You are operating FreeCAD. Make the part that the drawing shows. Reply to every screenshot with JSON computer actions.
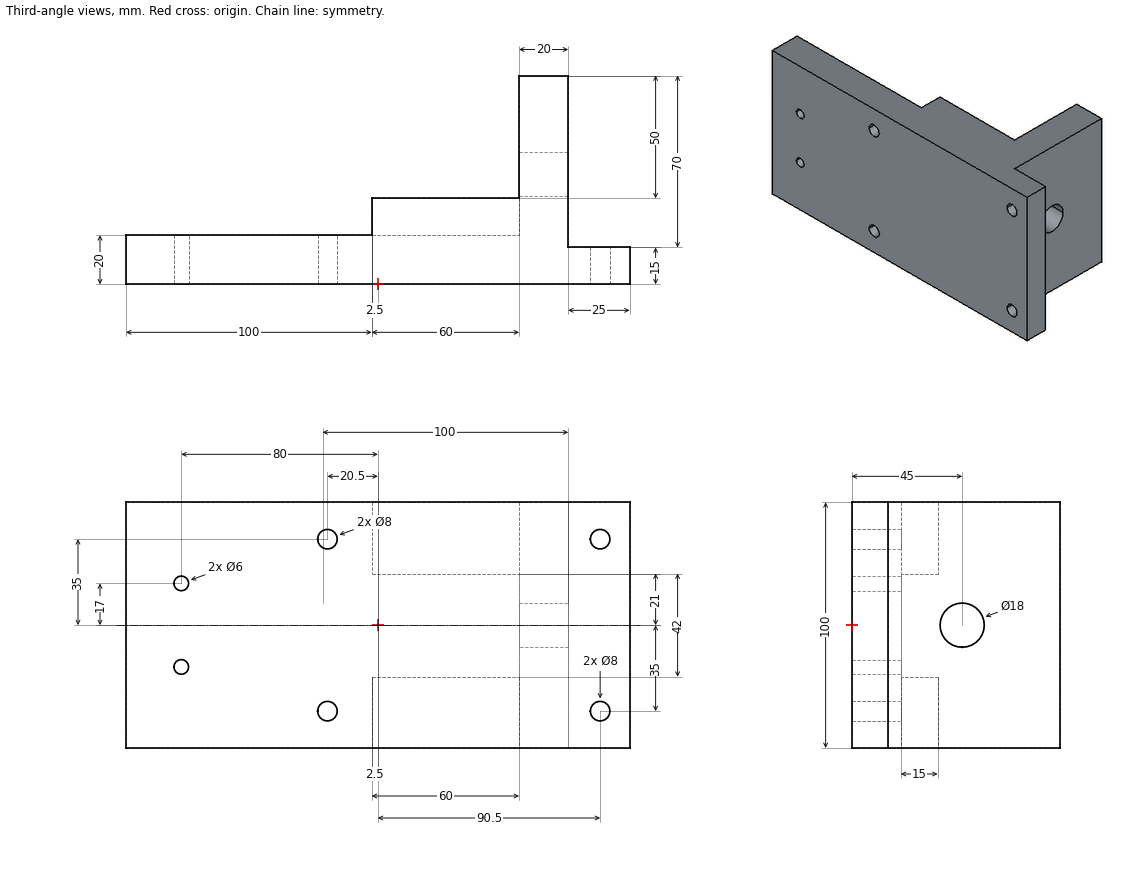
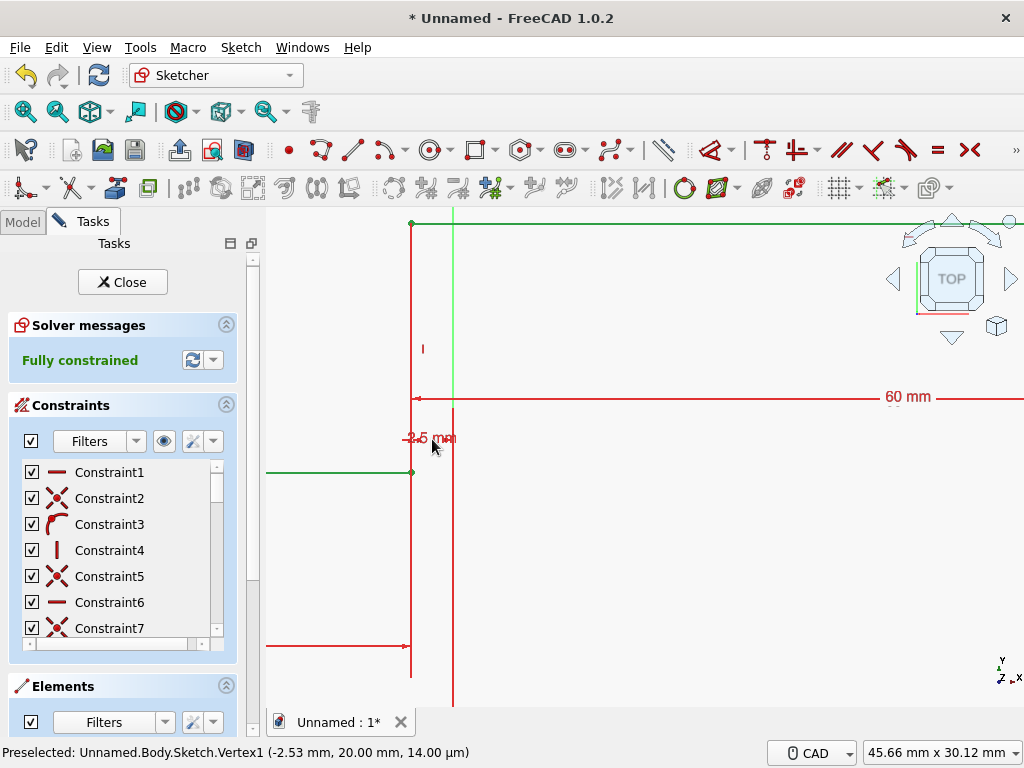
{"action": "left_click", "coordinate": [123, 282]}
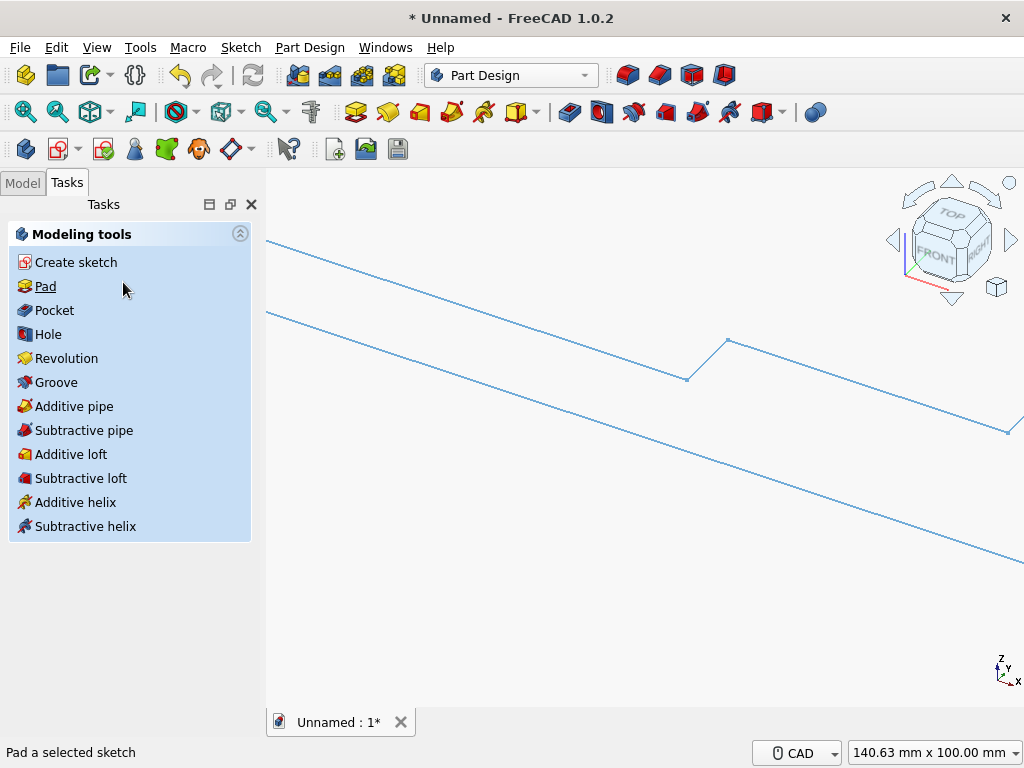
{"action": "left_click", "coordinate": [356, 112]}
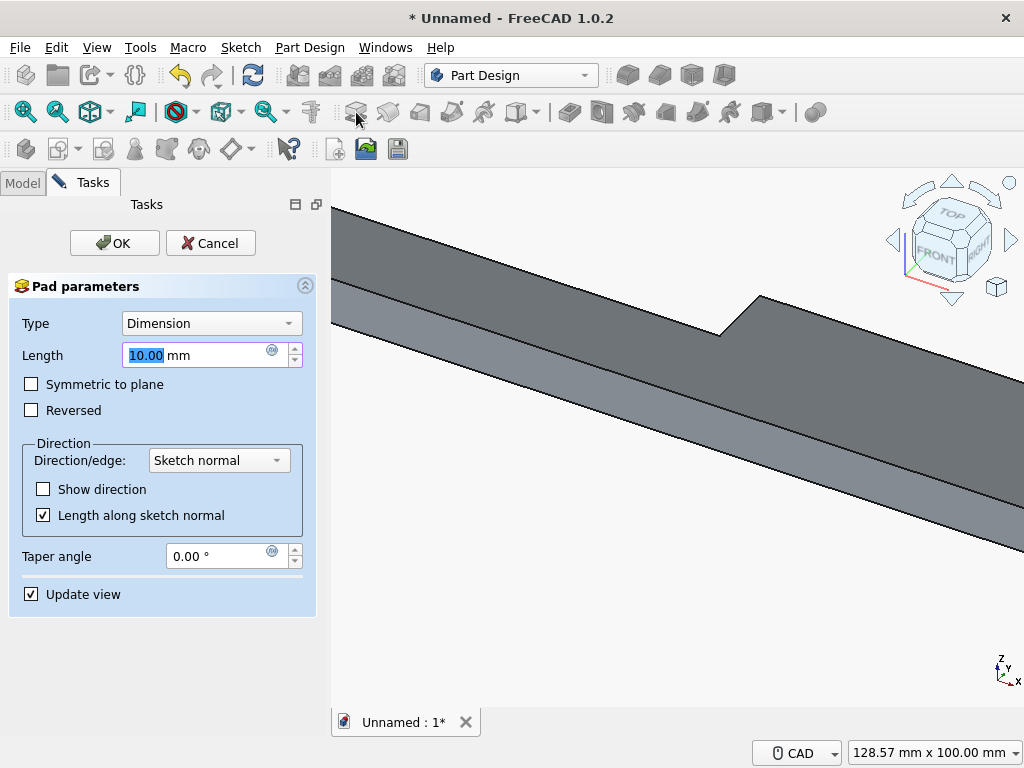
{"action": "type", "text": "100"}
{"action": "key", "text": "Tab"}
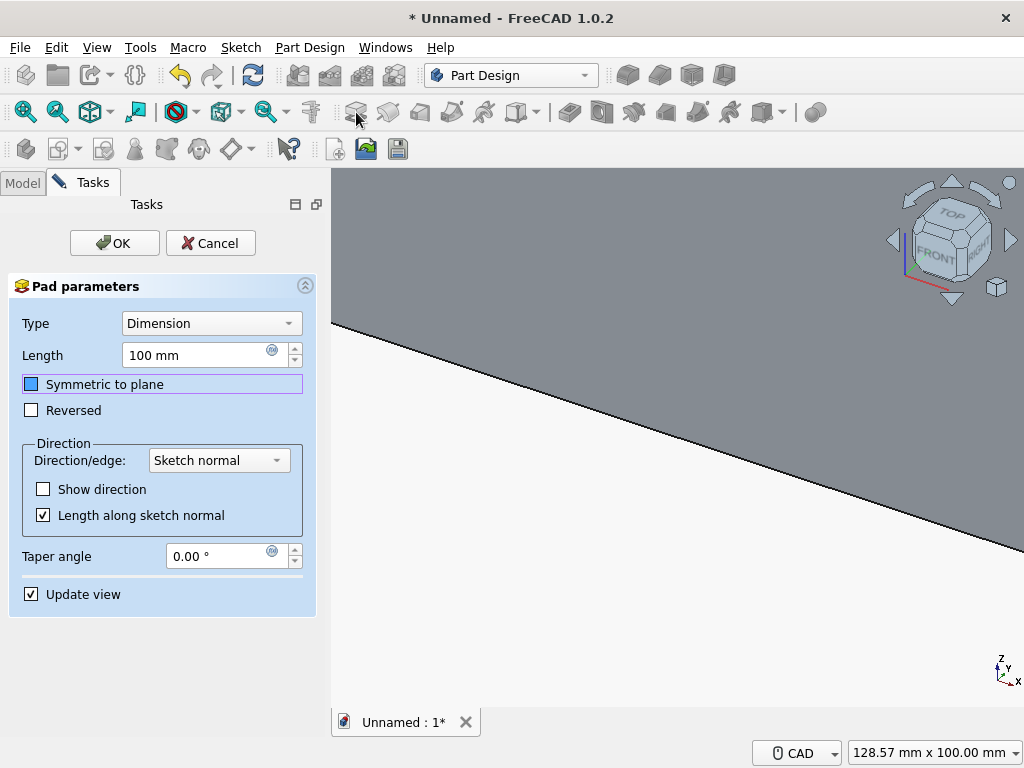
{"action": "left_click", "coordinate": [30, 384]}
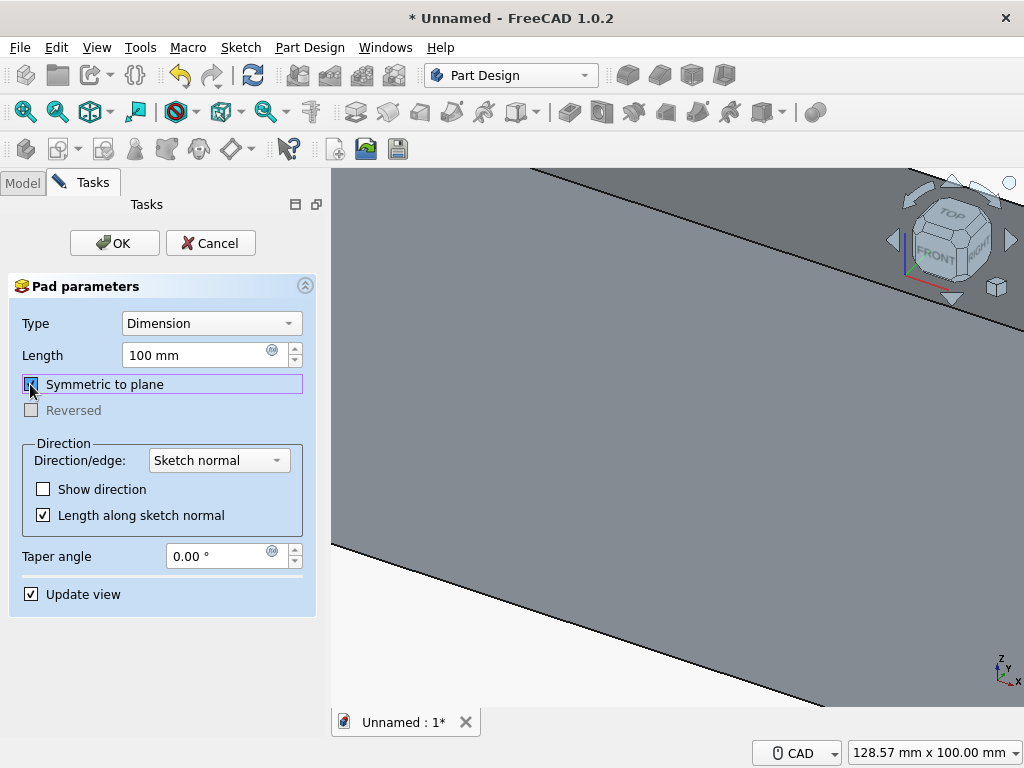
{"action": "left_click", "coordinate": [115, 243]}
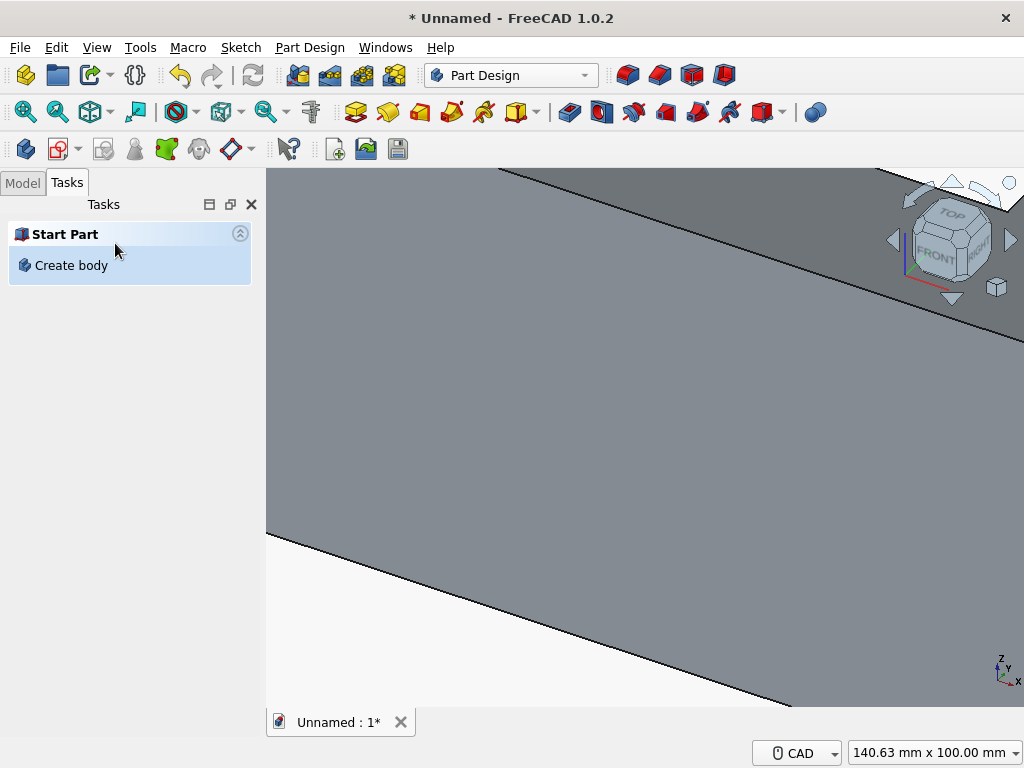
{"action": "left_click", "coordinate": [26, 112]}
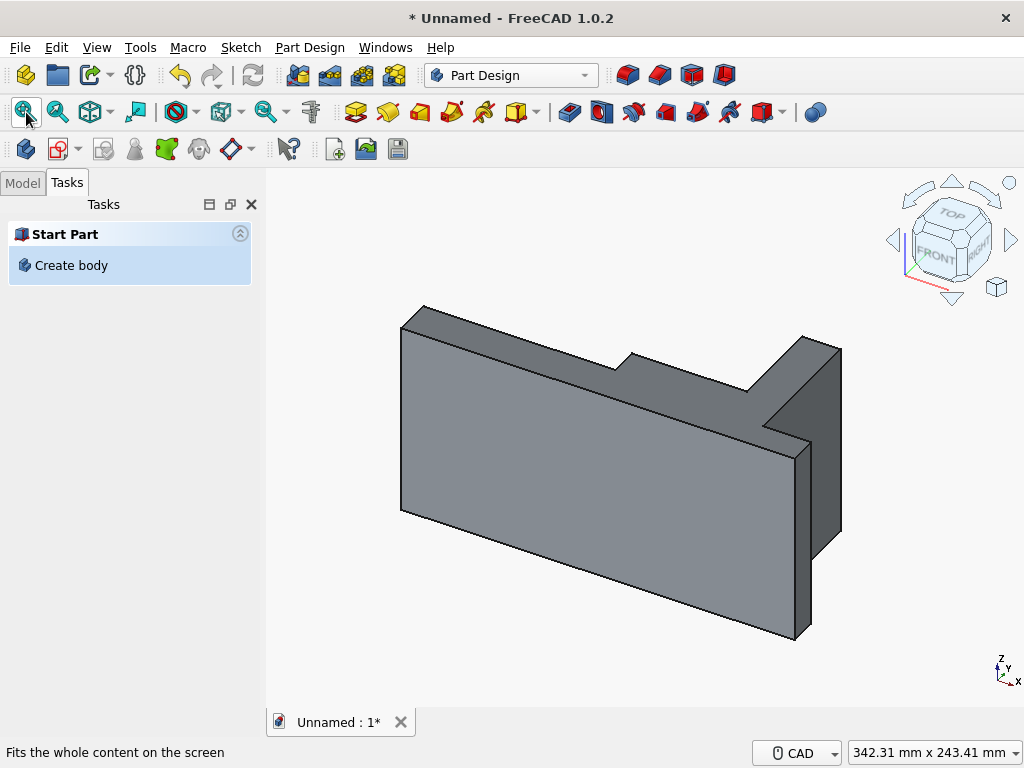
{"action": "key", "text": "4"}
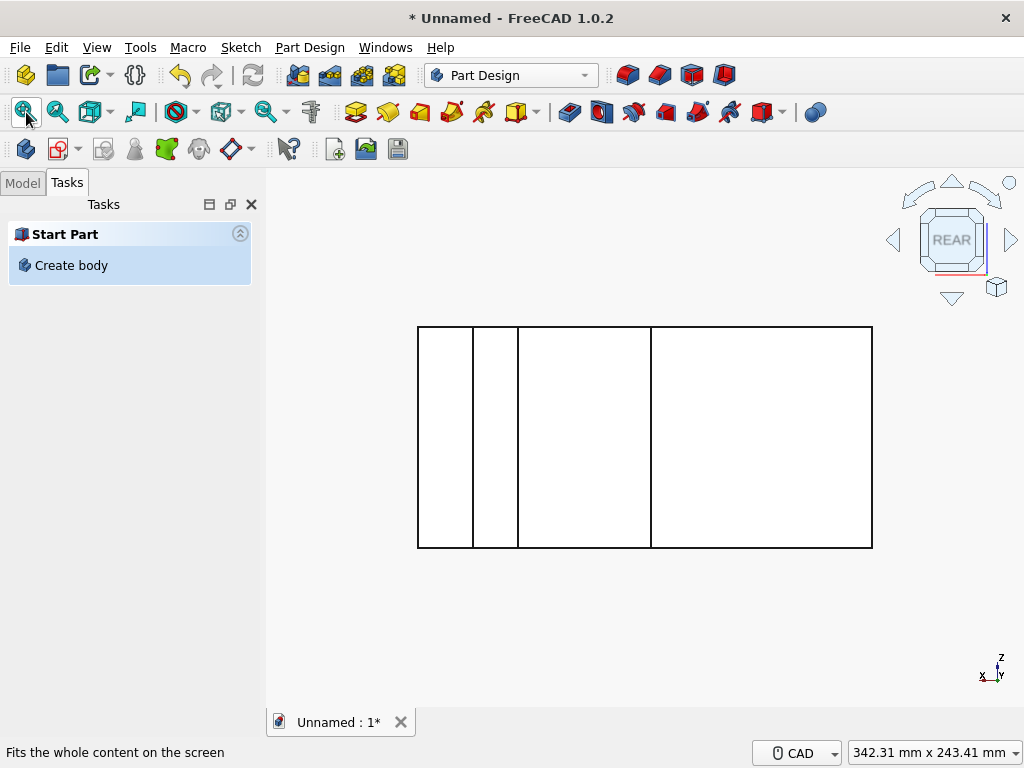
{"action": "left_click", "coordinate": [446, 373]}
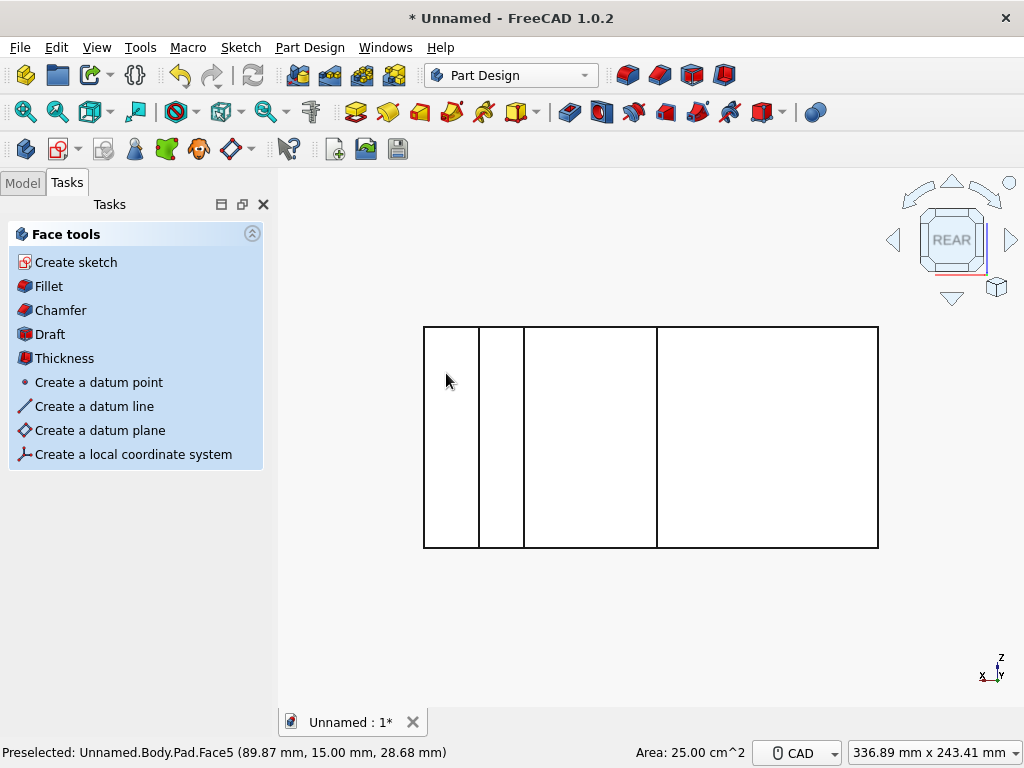
{"action": "left_click", "coordinate": [58, 150]}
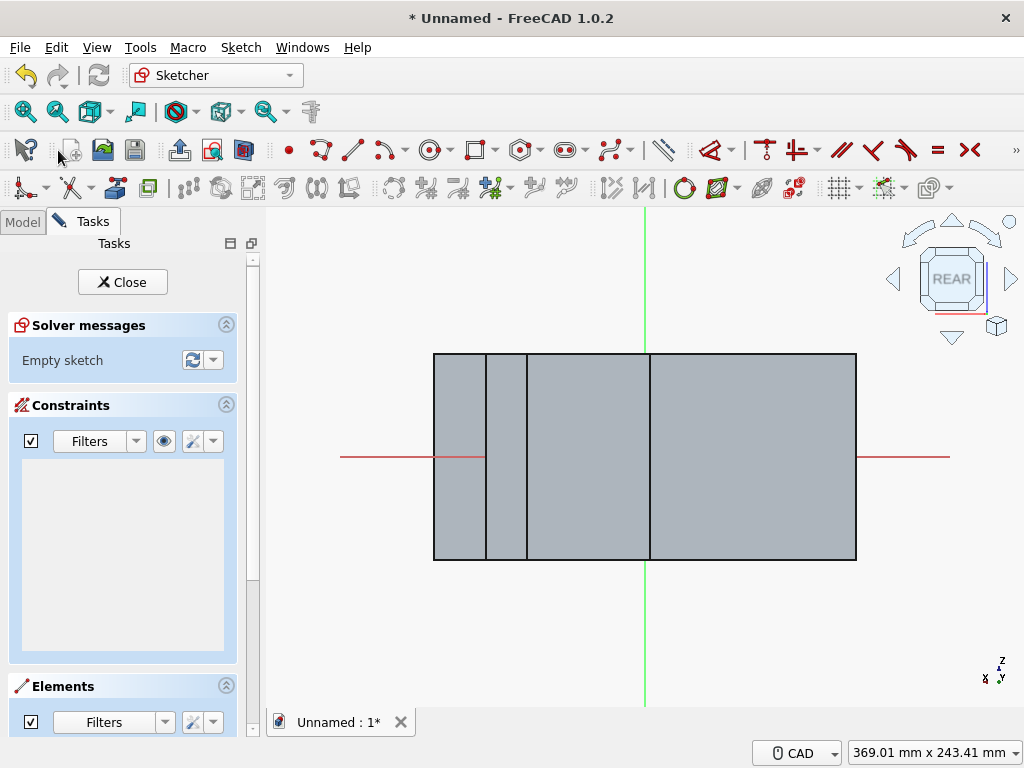
{"action": "left_click", "coordinate": [244, 150]}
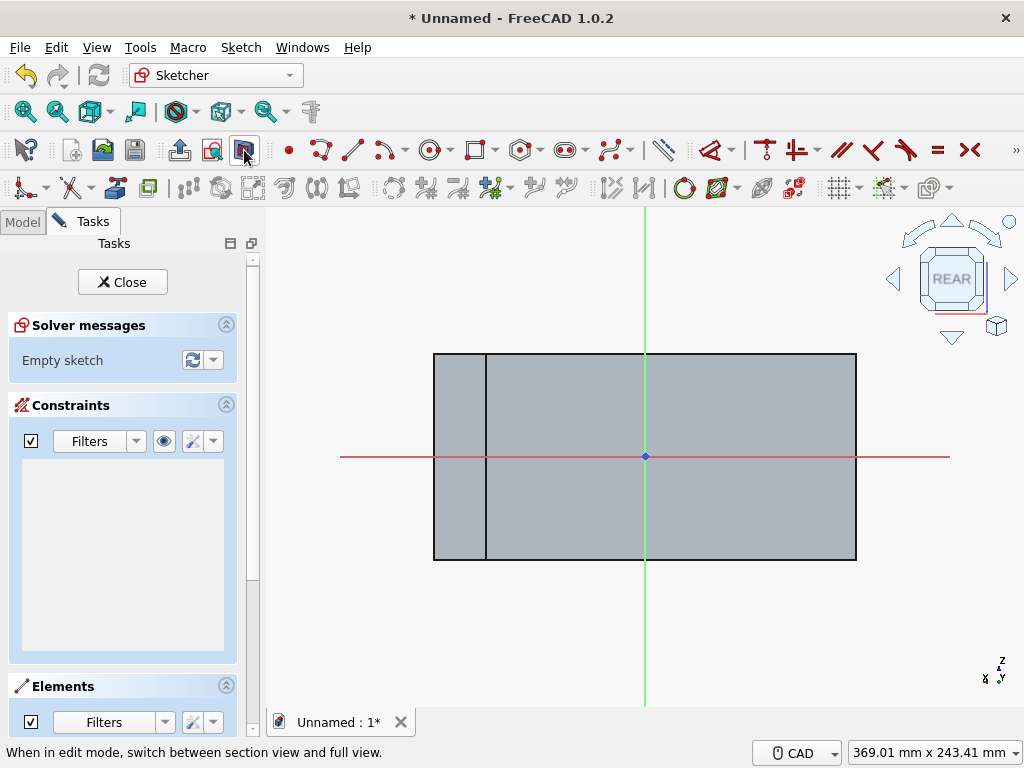
{"action": "scroll", "coordinate": [513, 457], "scroll_direction": "up", "scroll_amount": 3}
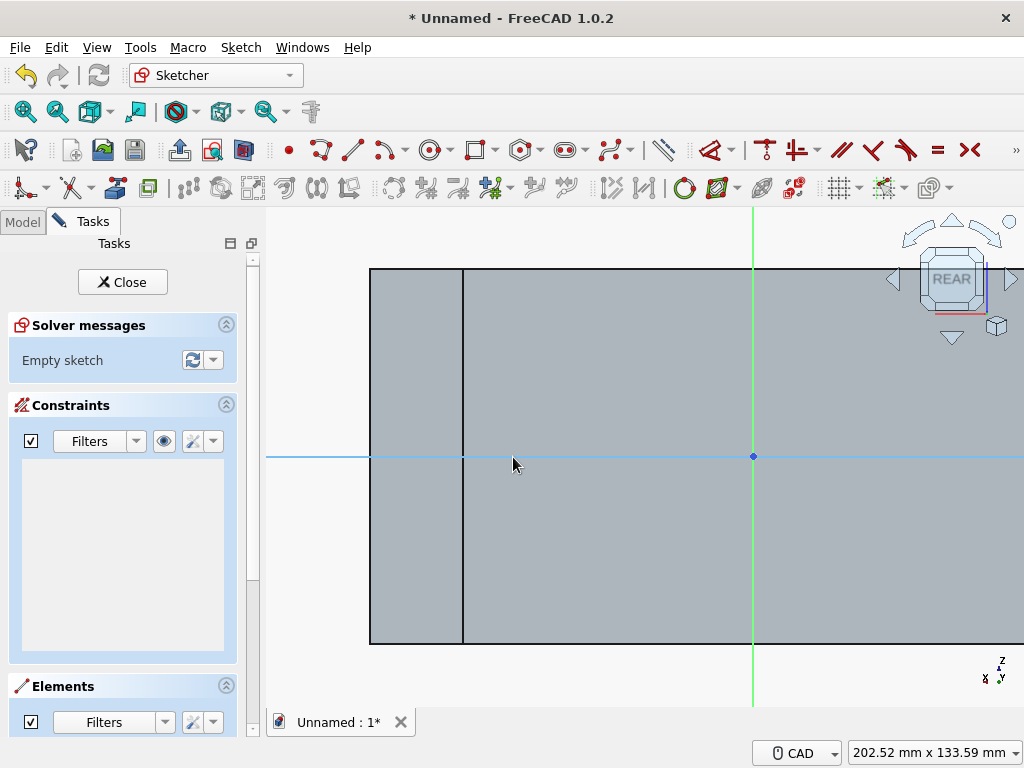
{"action": "left_click", "coordinate": [430, 150]}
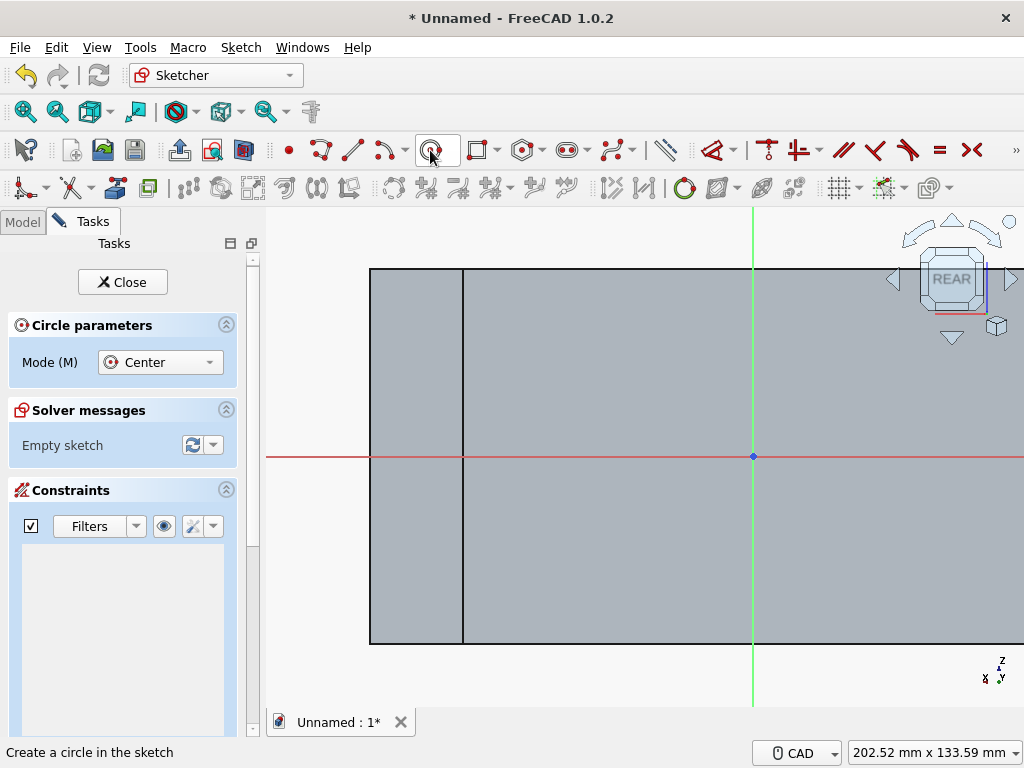
{"action": "scroll", "coordinate": [415, 588], "scroll_direction": "up", "scroll_amount": 3}